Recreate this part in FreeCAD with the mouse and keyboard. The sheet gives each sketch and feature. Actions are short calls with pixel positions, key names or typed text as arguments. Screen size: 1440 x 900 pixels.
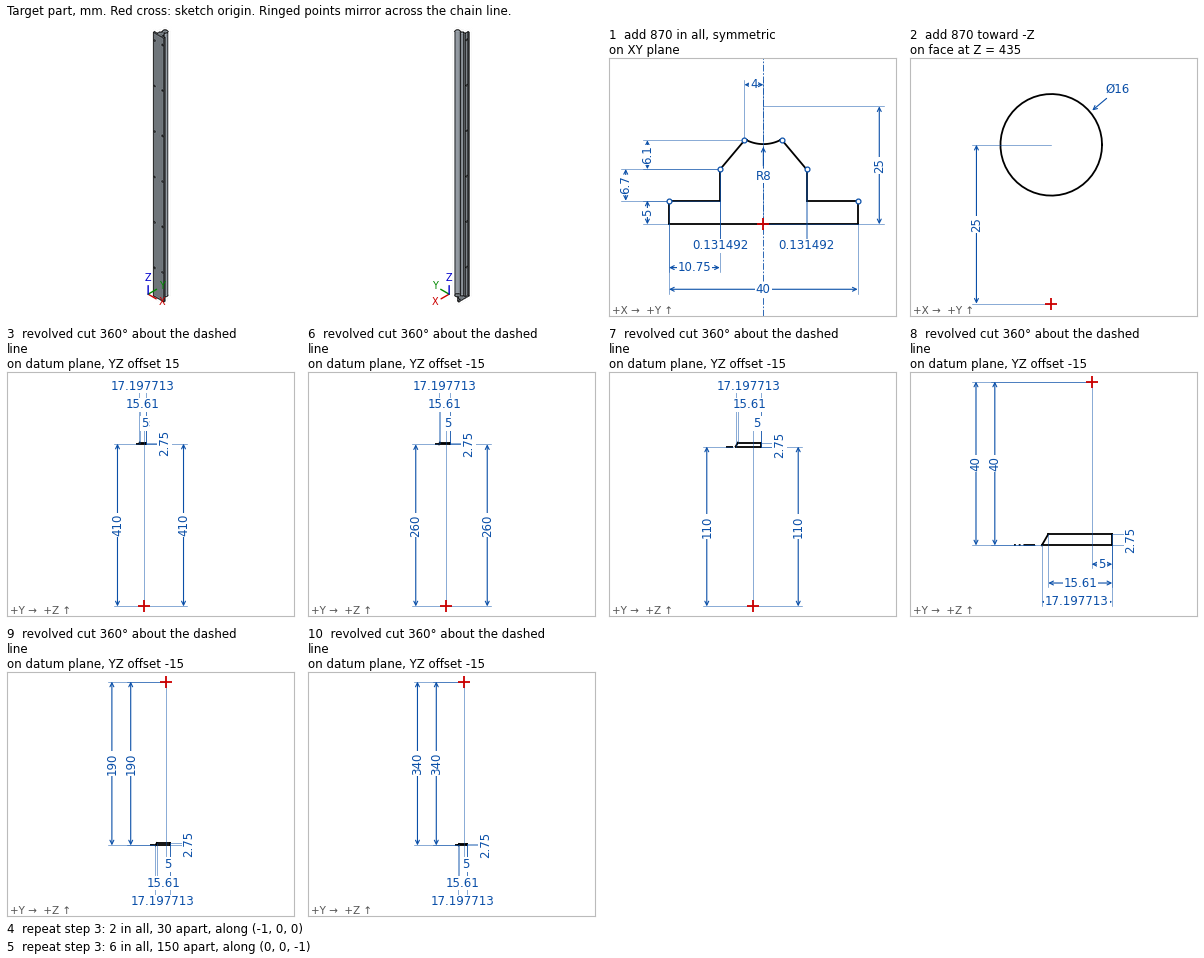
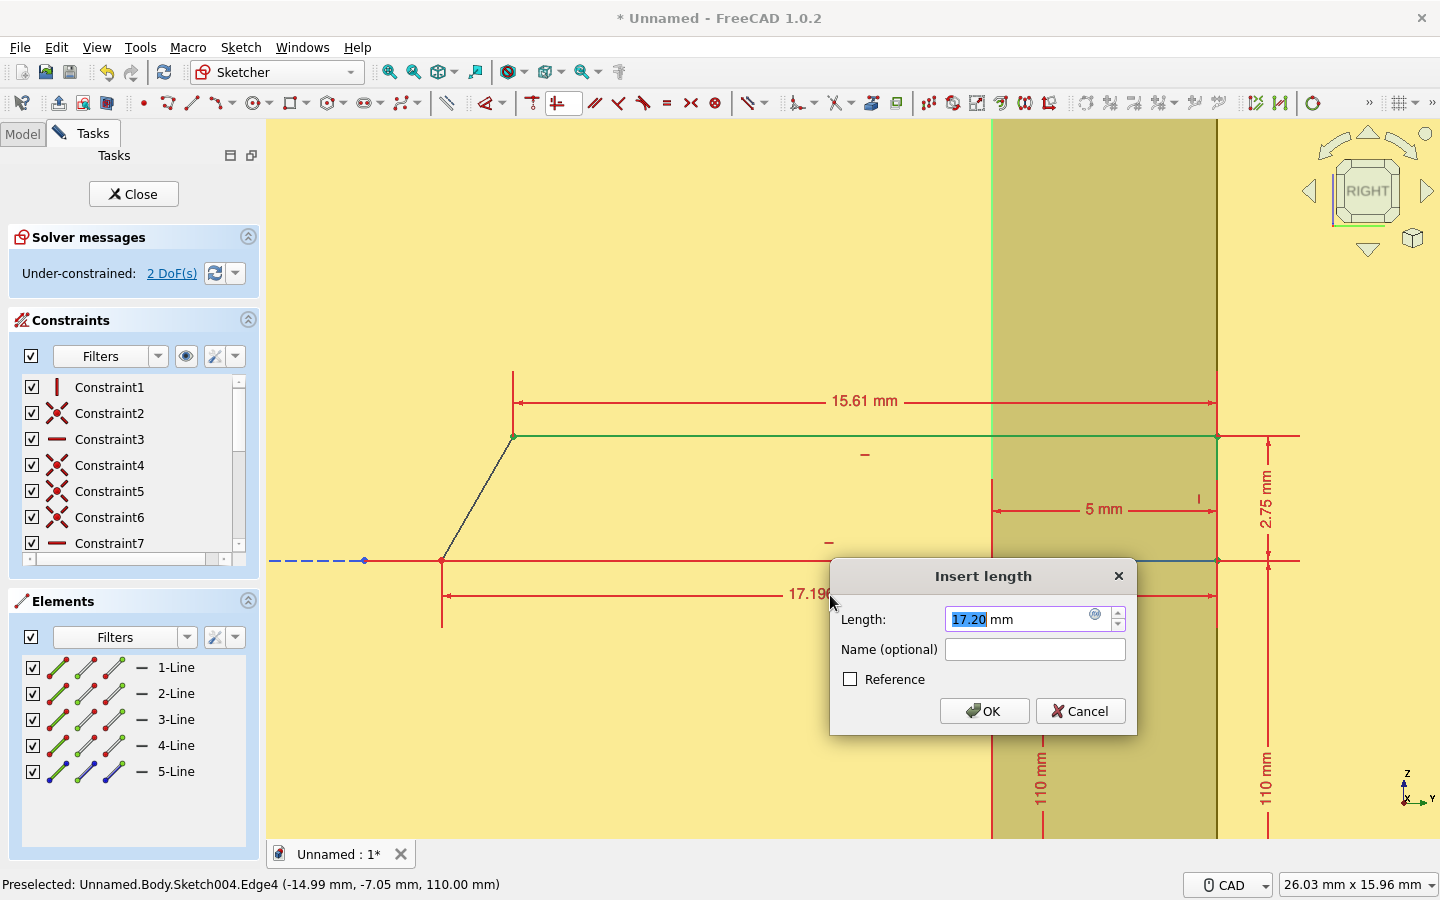
text(17.197713)
key(Return)
key(Escape)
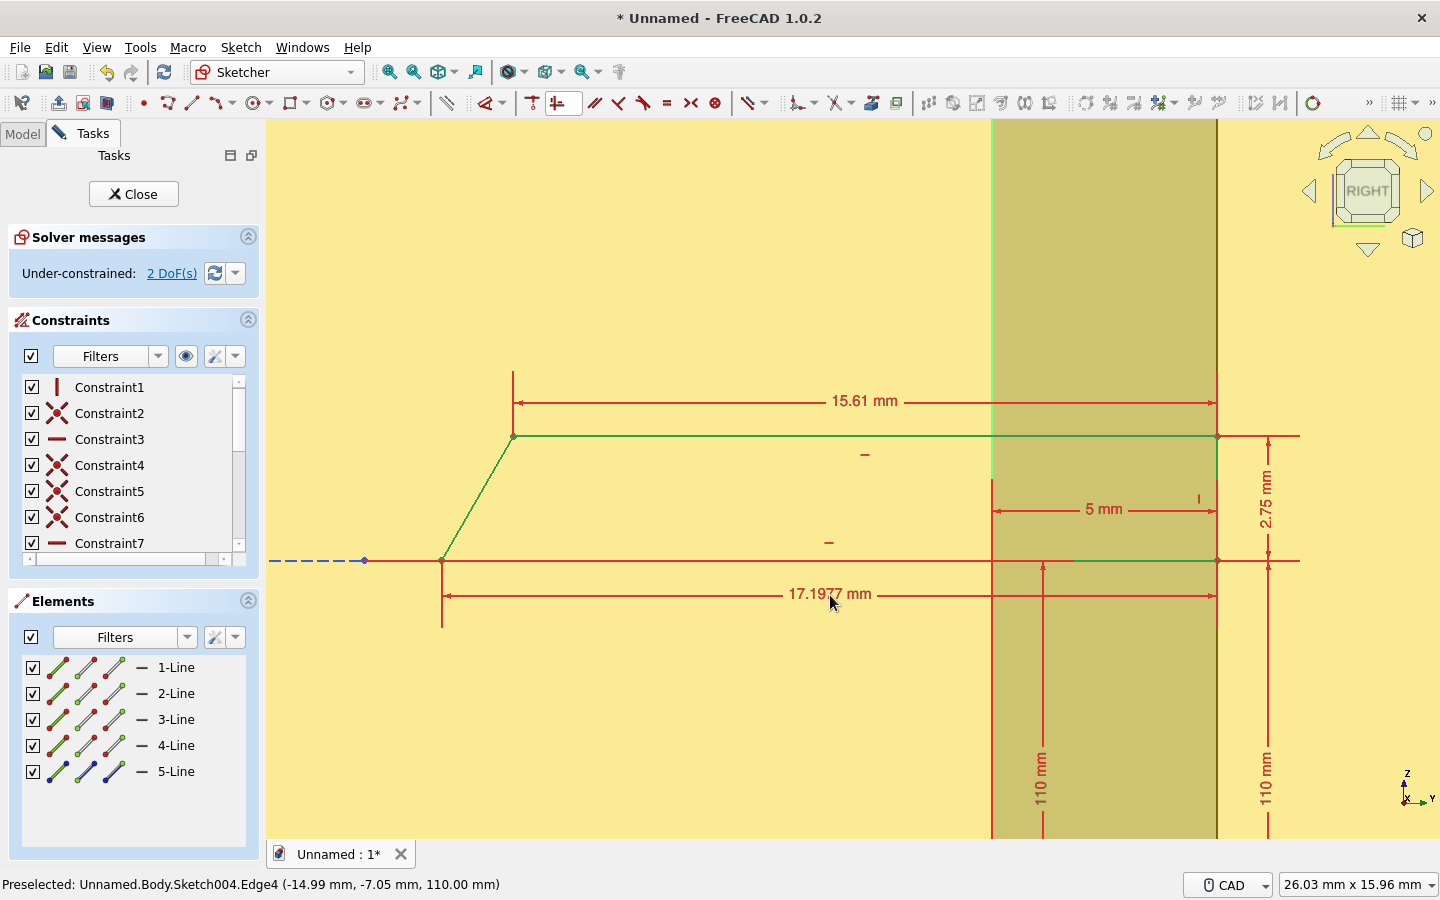
click(134, 194)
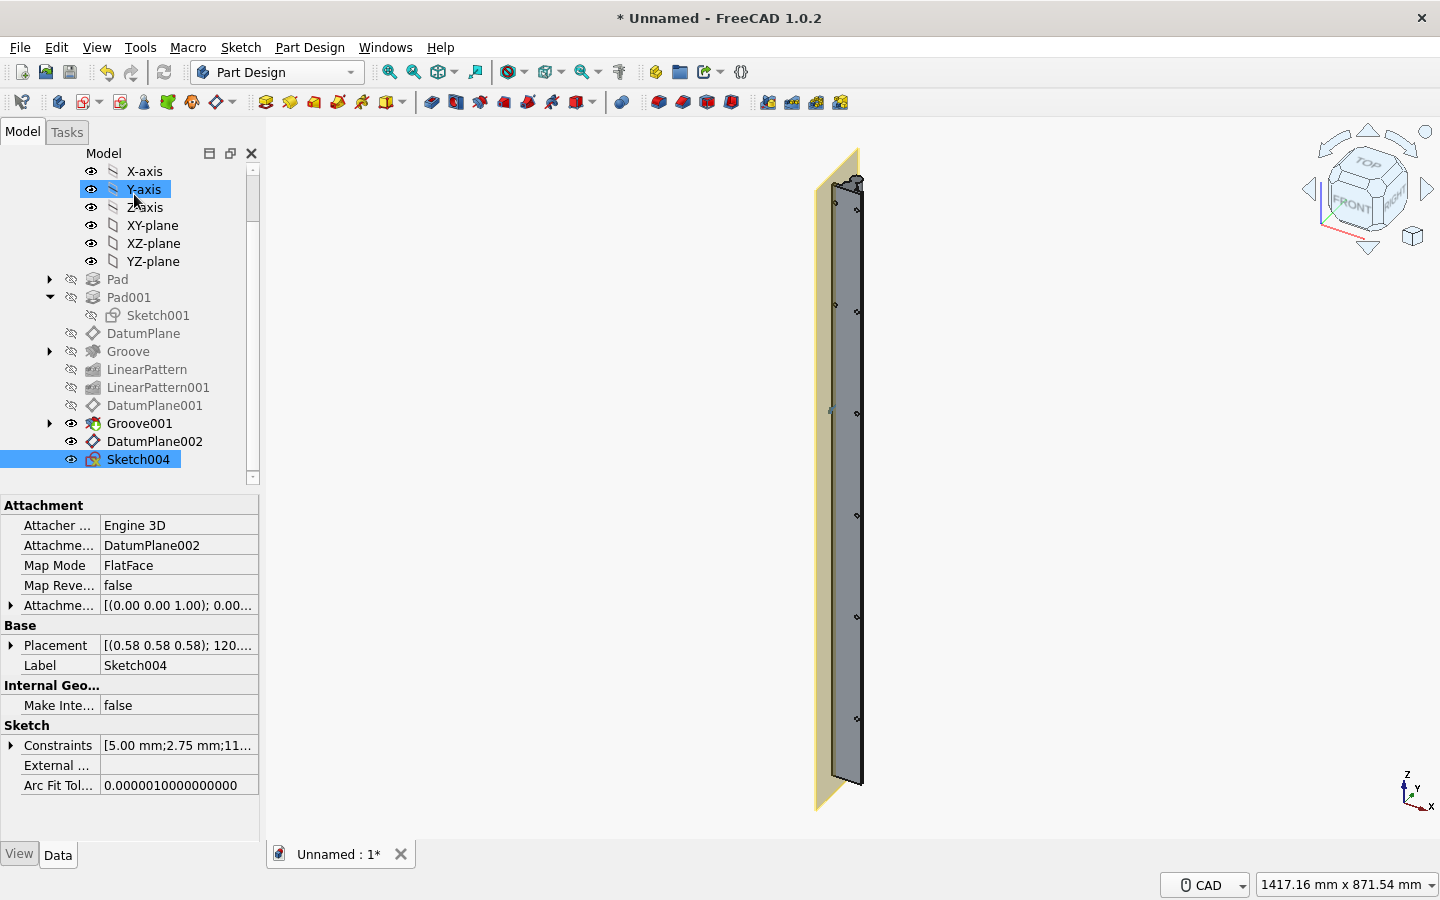
click(480, 102)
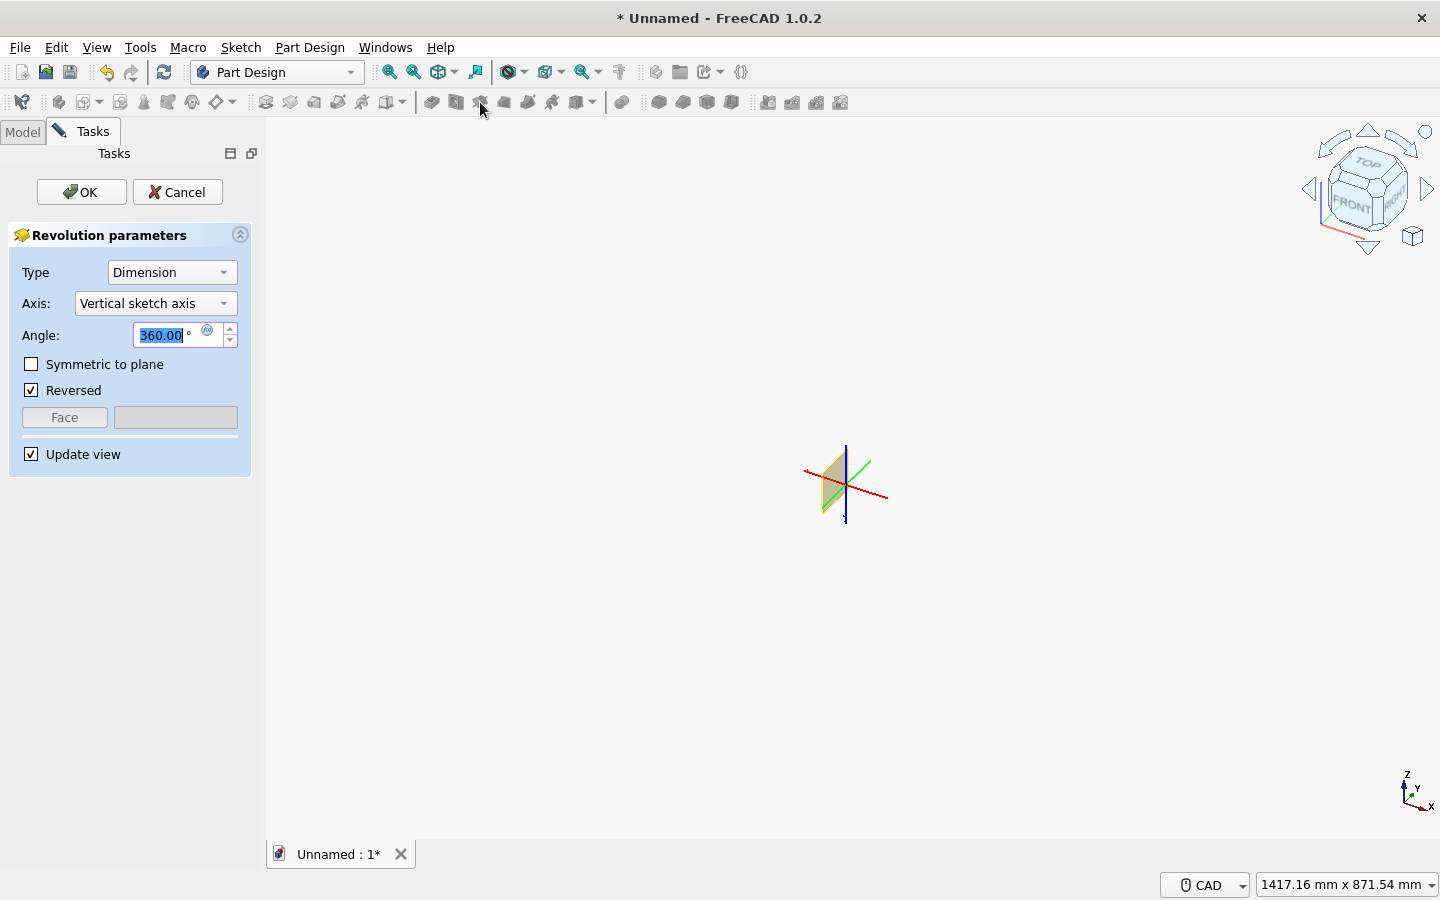
click(156, 304)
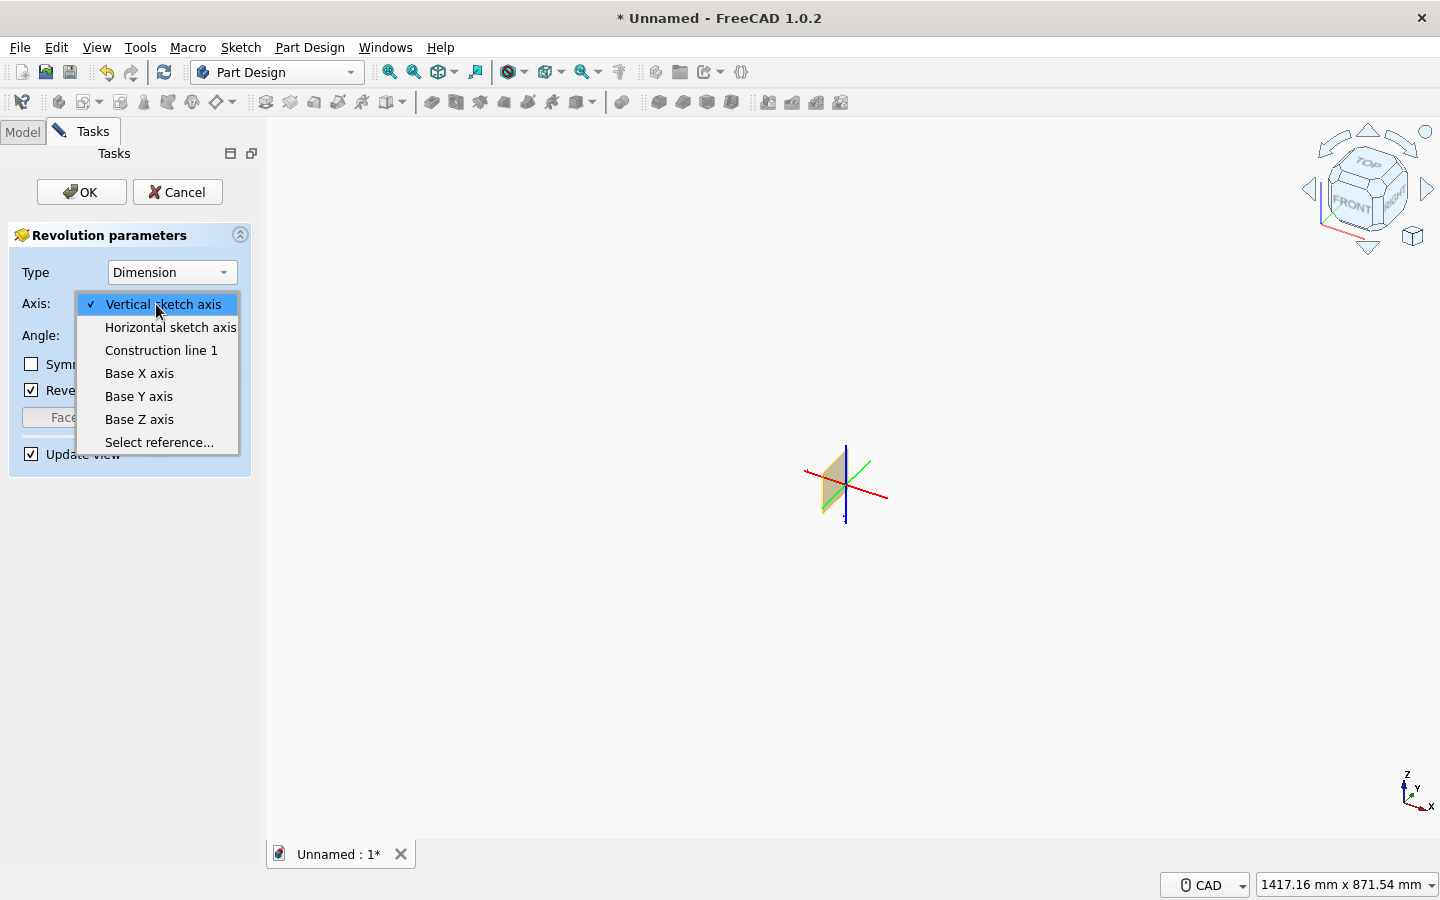
click(156, 350)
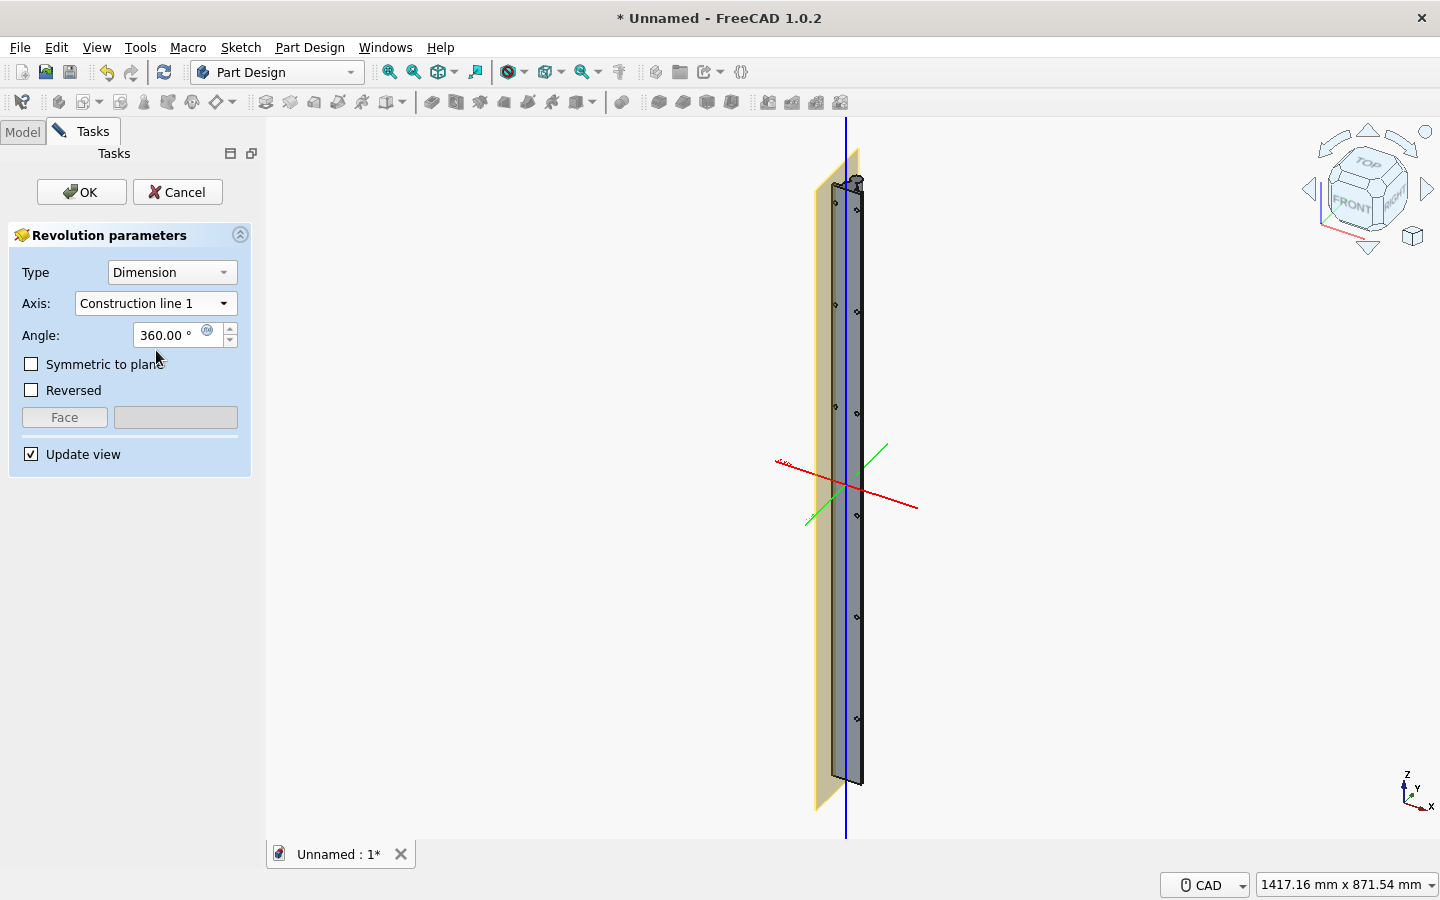
click(82, 192)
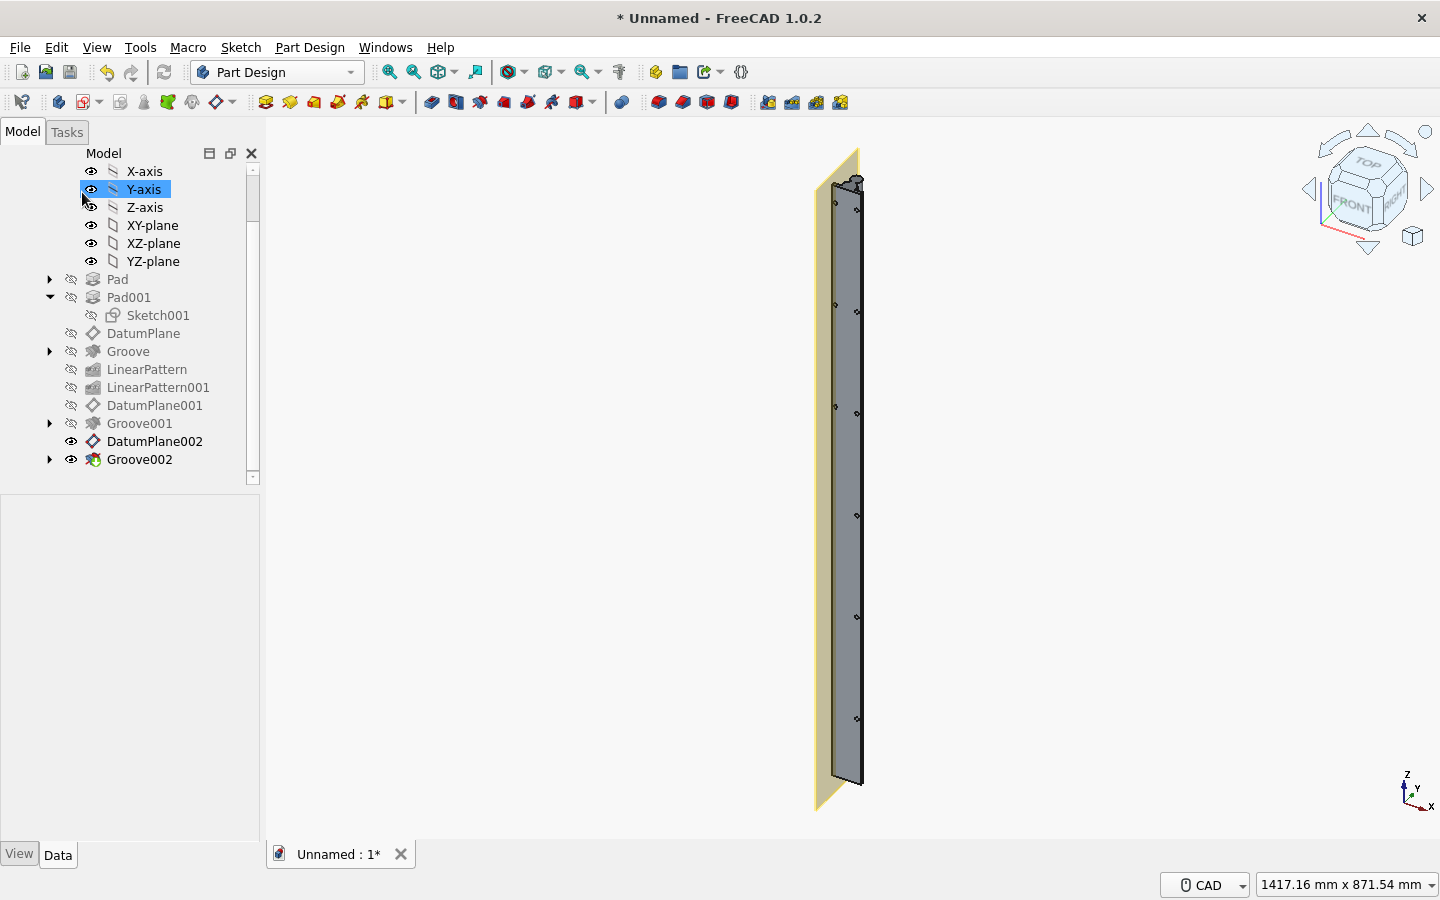
click(116, 441)
key(space)